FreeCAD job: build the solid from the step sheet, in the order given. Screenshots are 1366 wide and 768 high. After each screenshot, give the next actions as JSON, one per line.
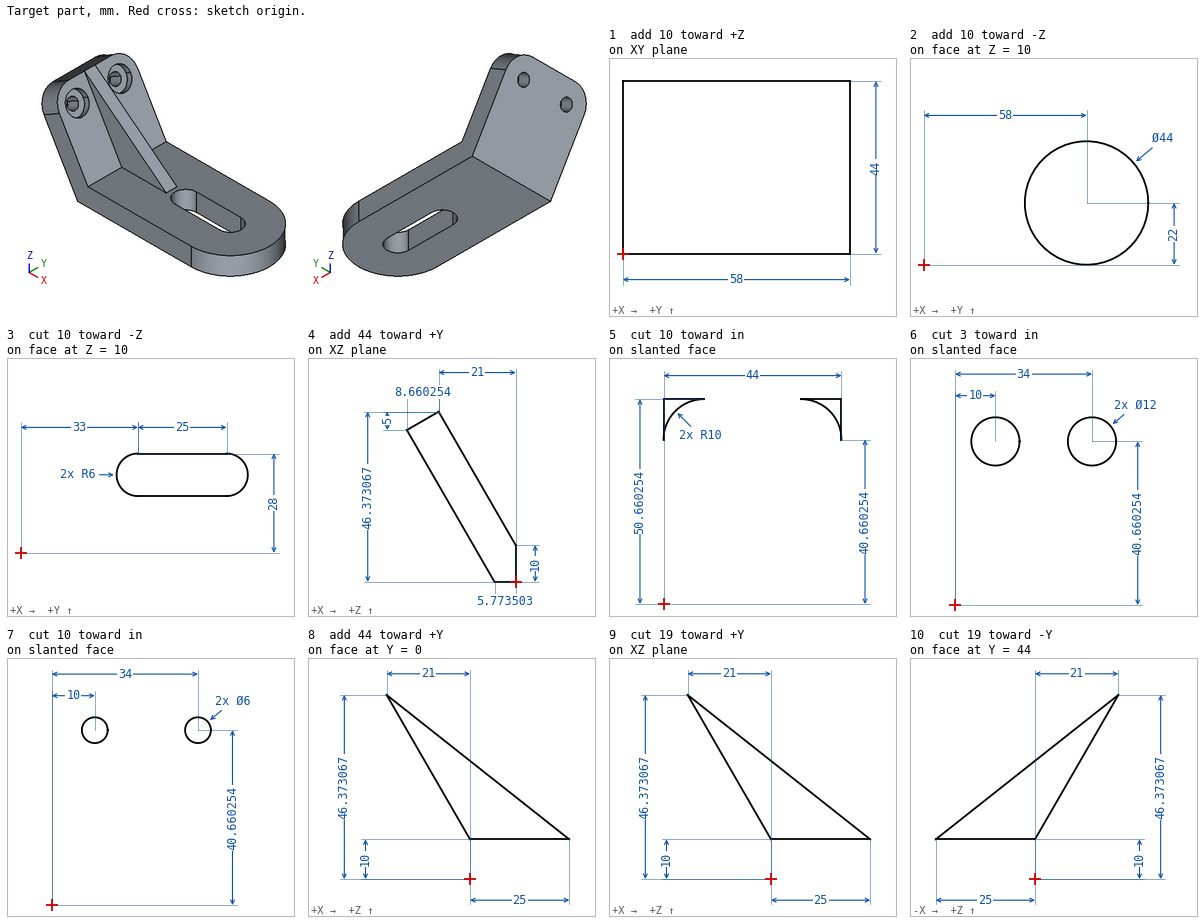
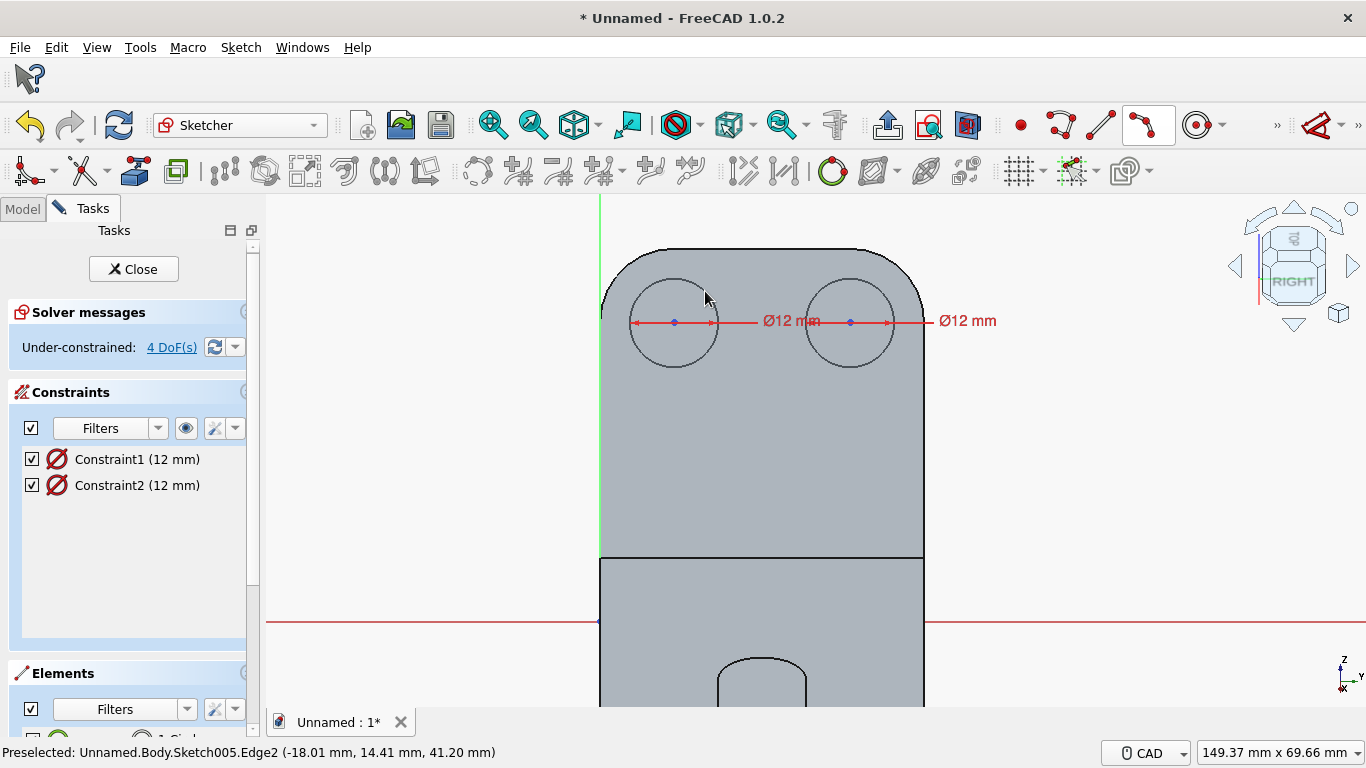
{"action": "left_click", "coordinate": [850, 323]}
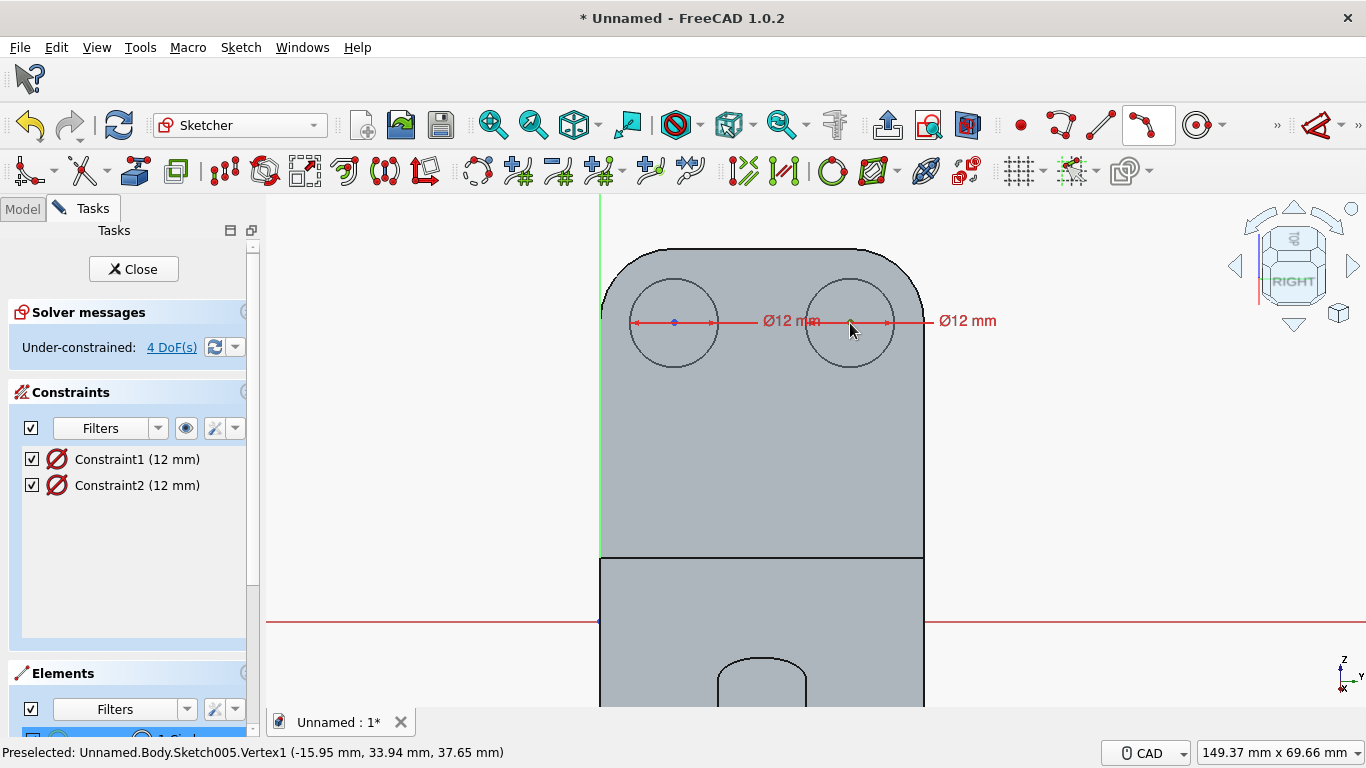
{"action": "left_click", "coordinate": [674, 323]}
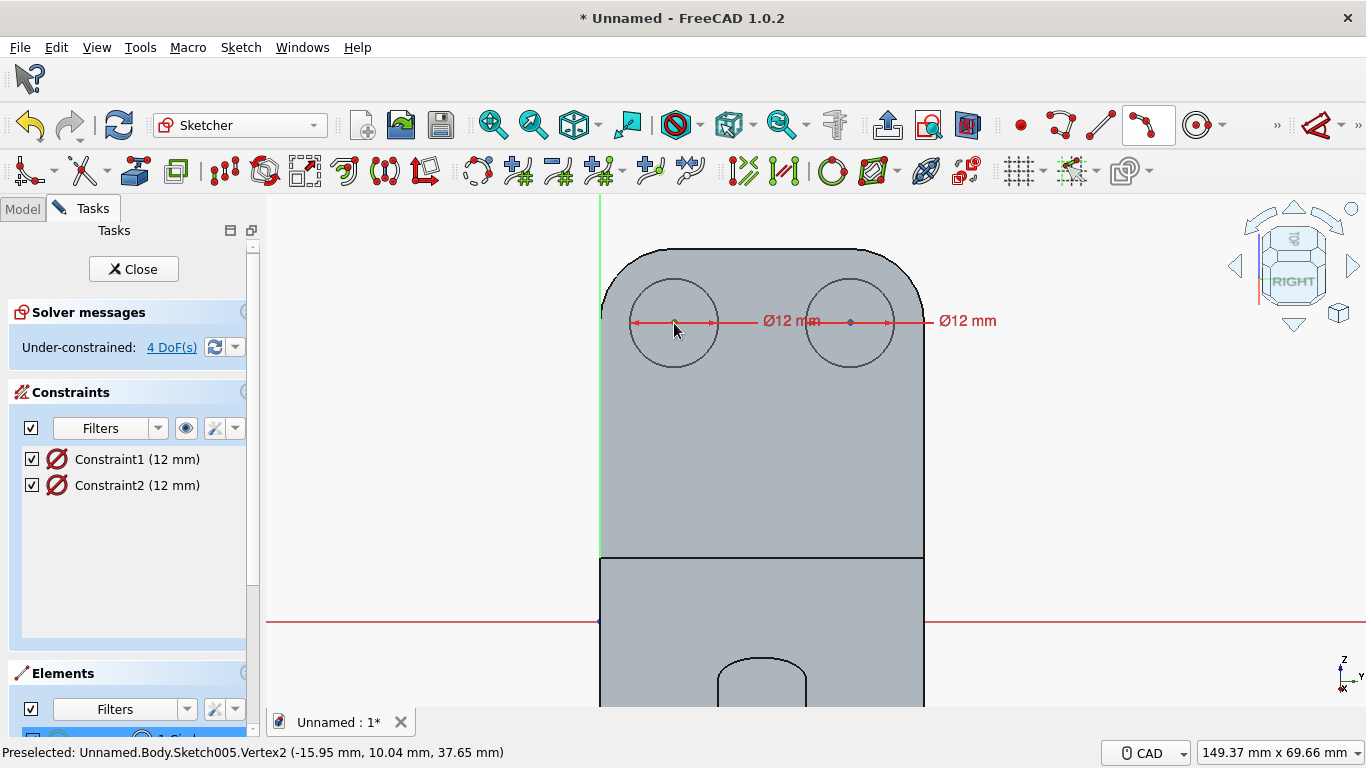
{"action": "key", "text": "h"}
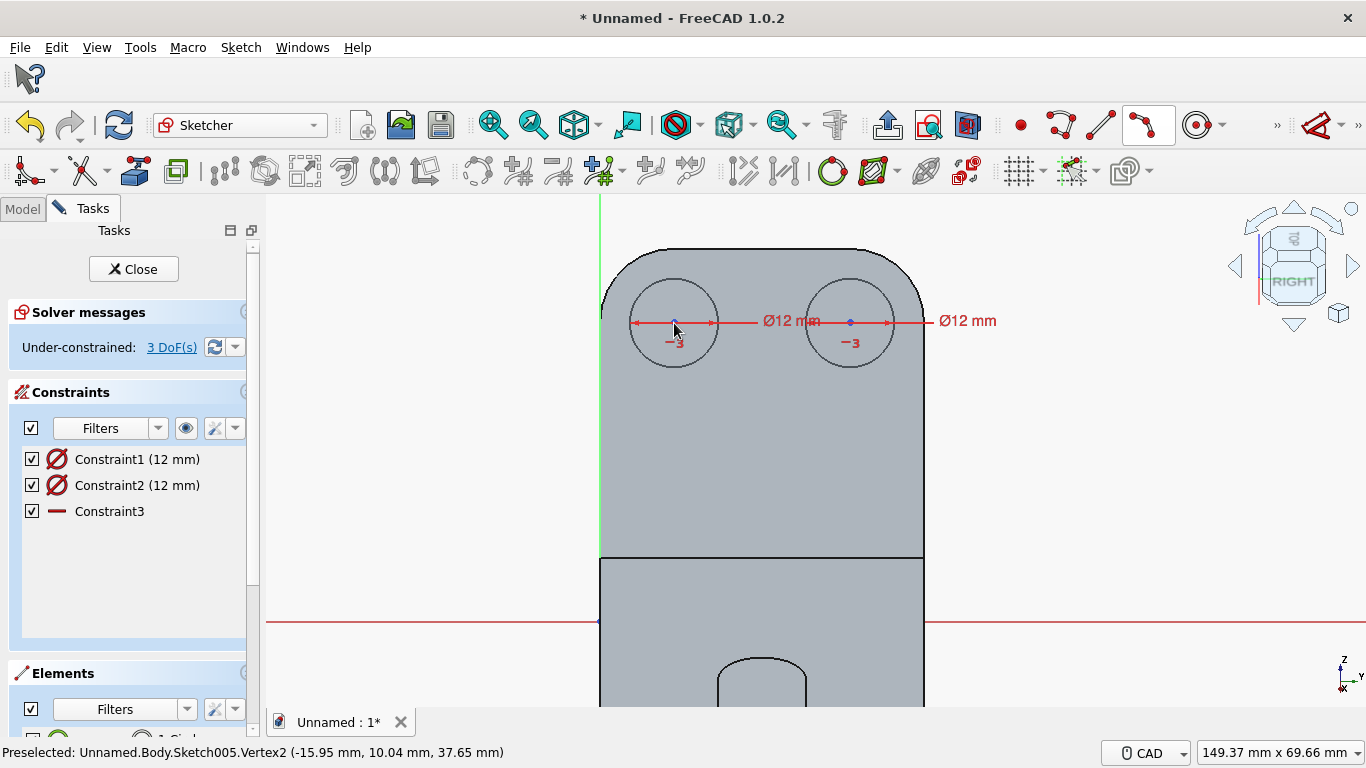
{"action": "left_click", "coordinate": [1316, 126]}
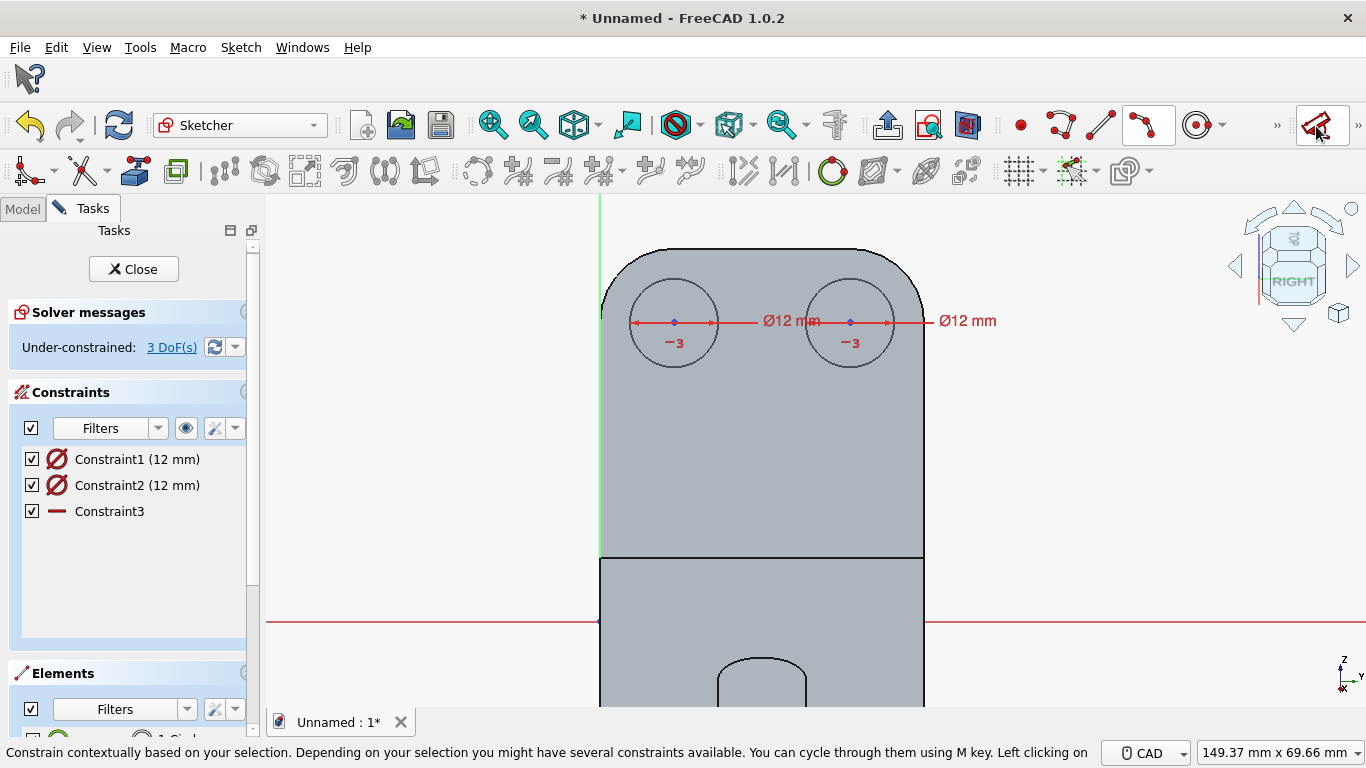
{"action": "left_click", "coordinate": [850, 323]}
{"action": "left_click", "coordinate": [725, 656]}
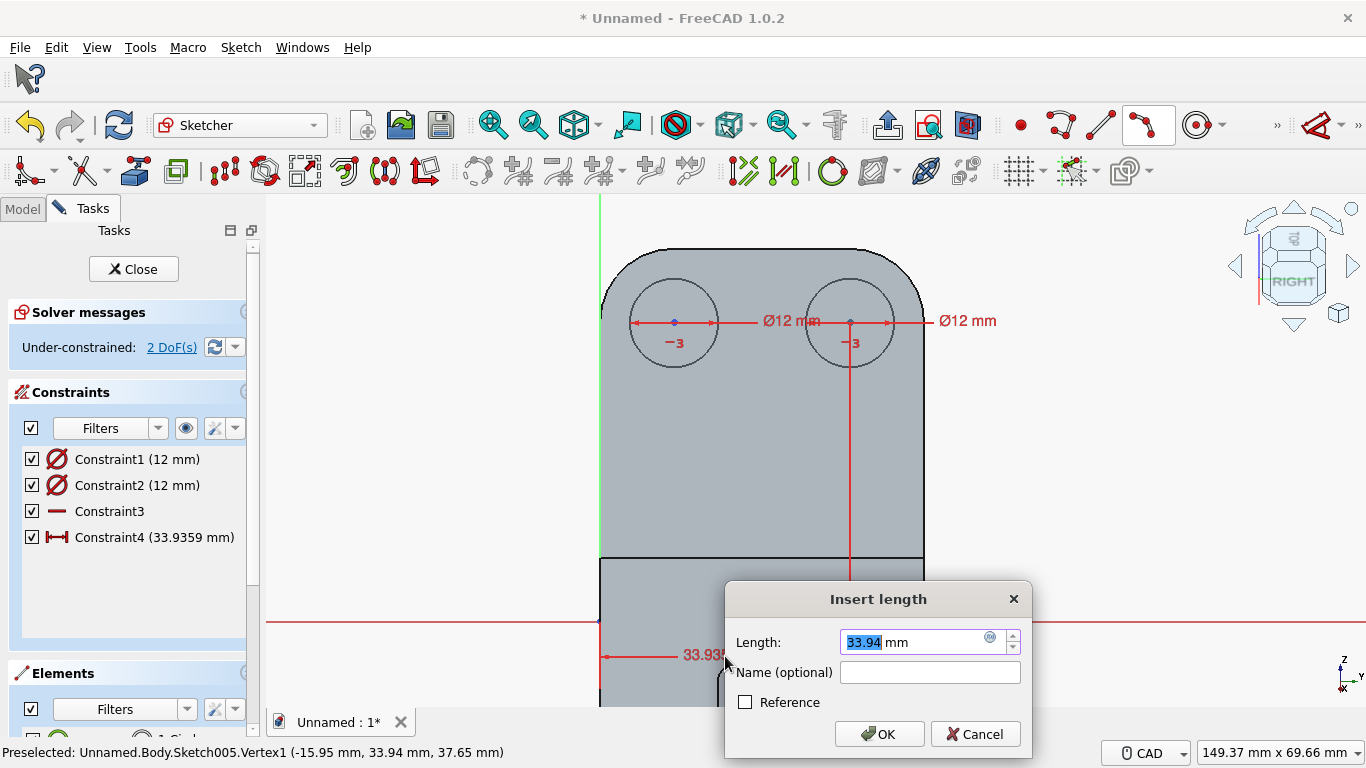
{"action": "type", "text": "34"}
{"action": "key", "text": "Return"}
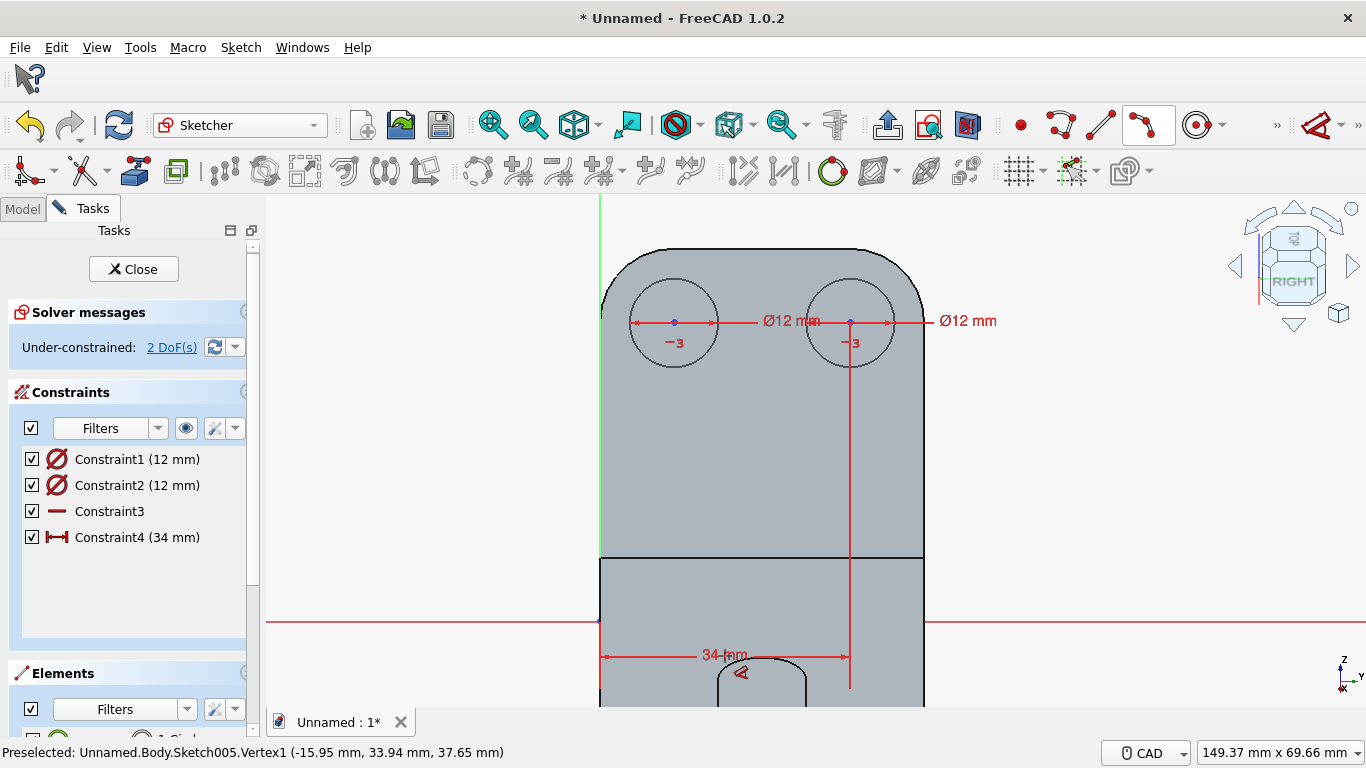
{"action": "left_click", "coordinate": [674, 323]}
{"action": "left_click", "coordinate": [637, 656]}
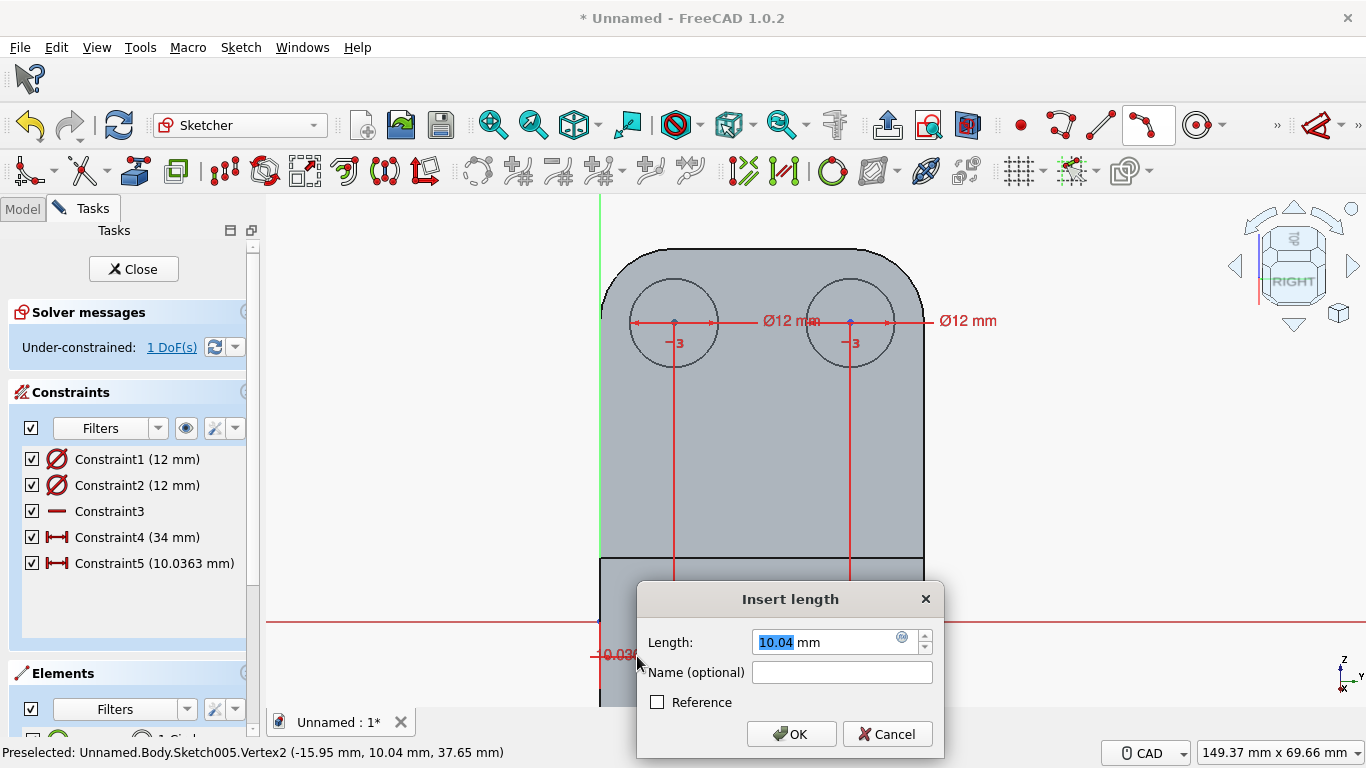
{"action": "type", "text": "10"}
{"action": "key", "text": "Return"}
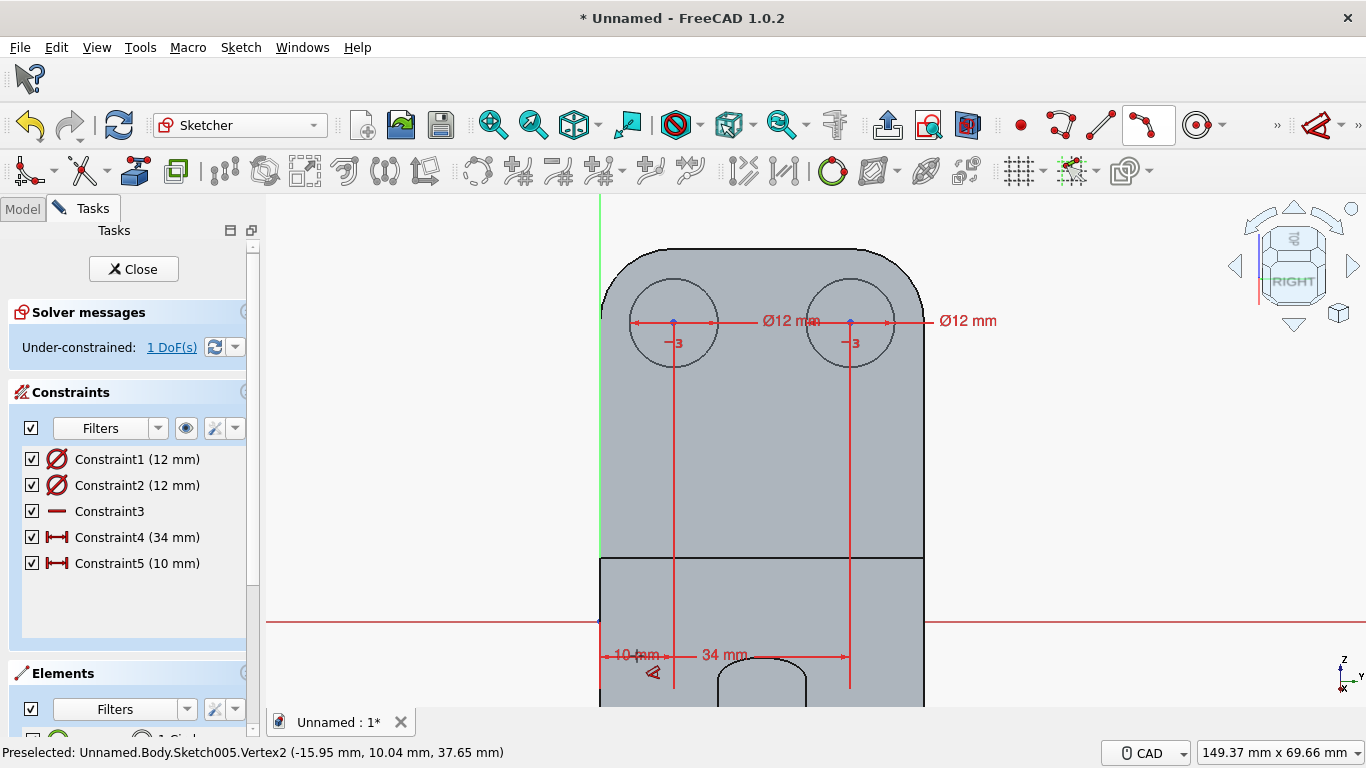
{"action": "left_click", "coordinate": [850, 323]}
{"action": "left_click", "coordinate": [566, 472]}